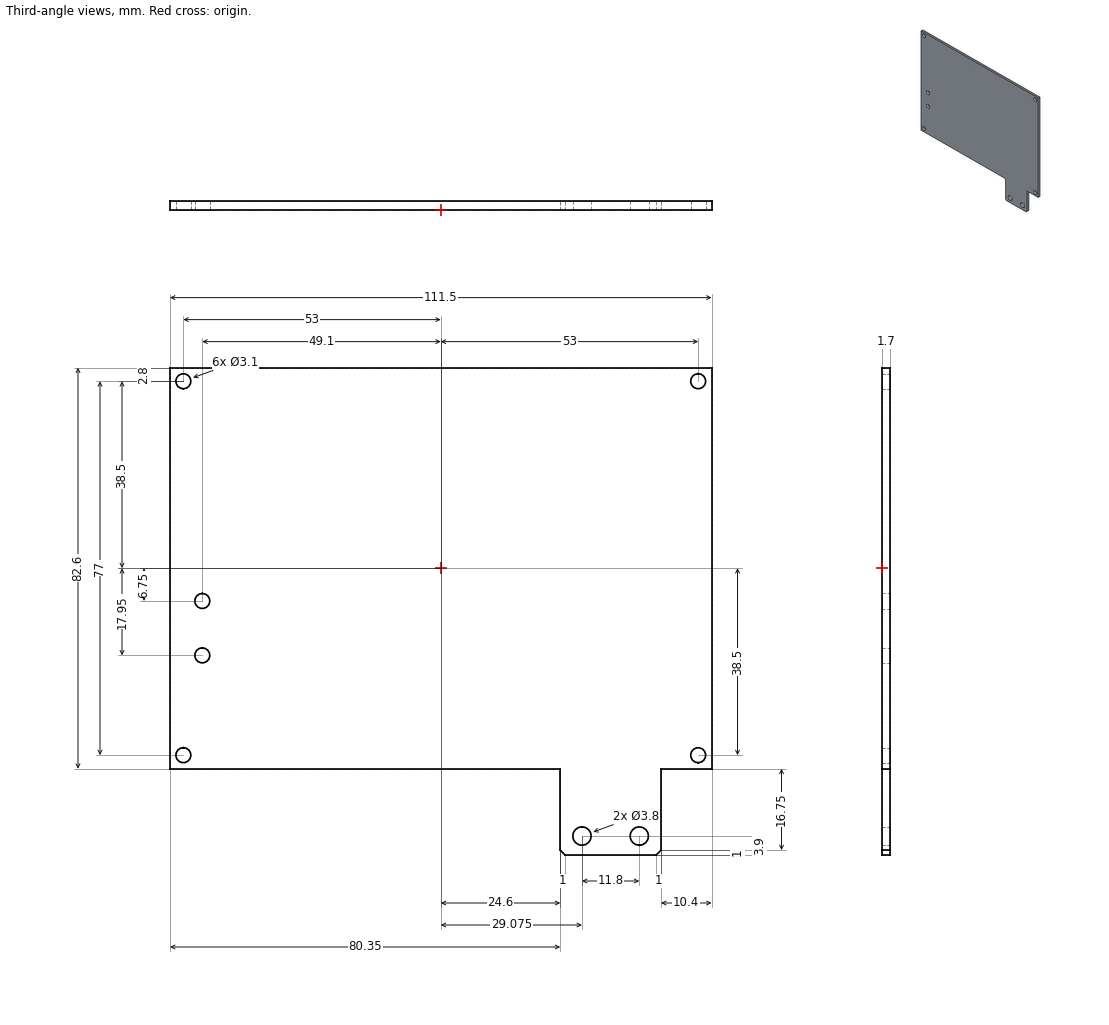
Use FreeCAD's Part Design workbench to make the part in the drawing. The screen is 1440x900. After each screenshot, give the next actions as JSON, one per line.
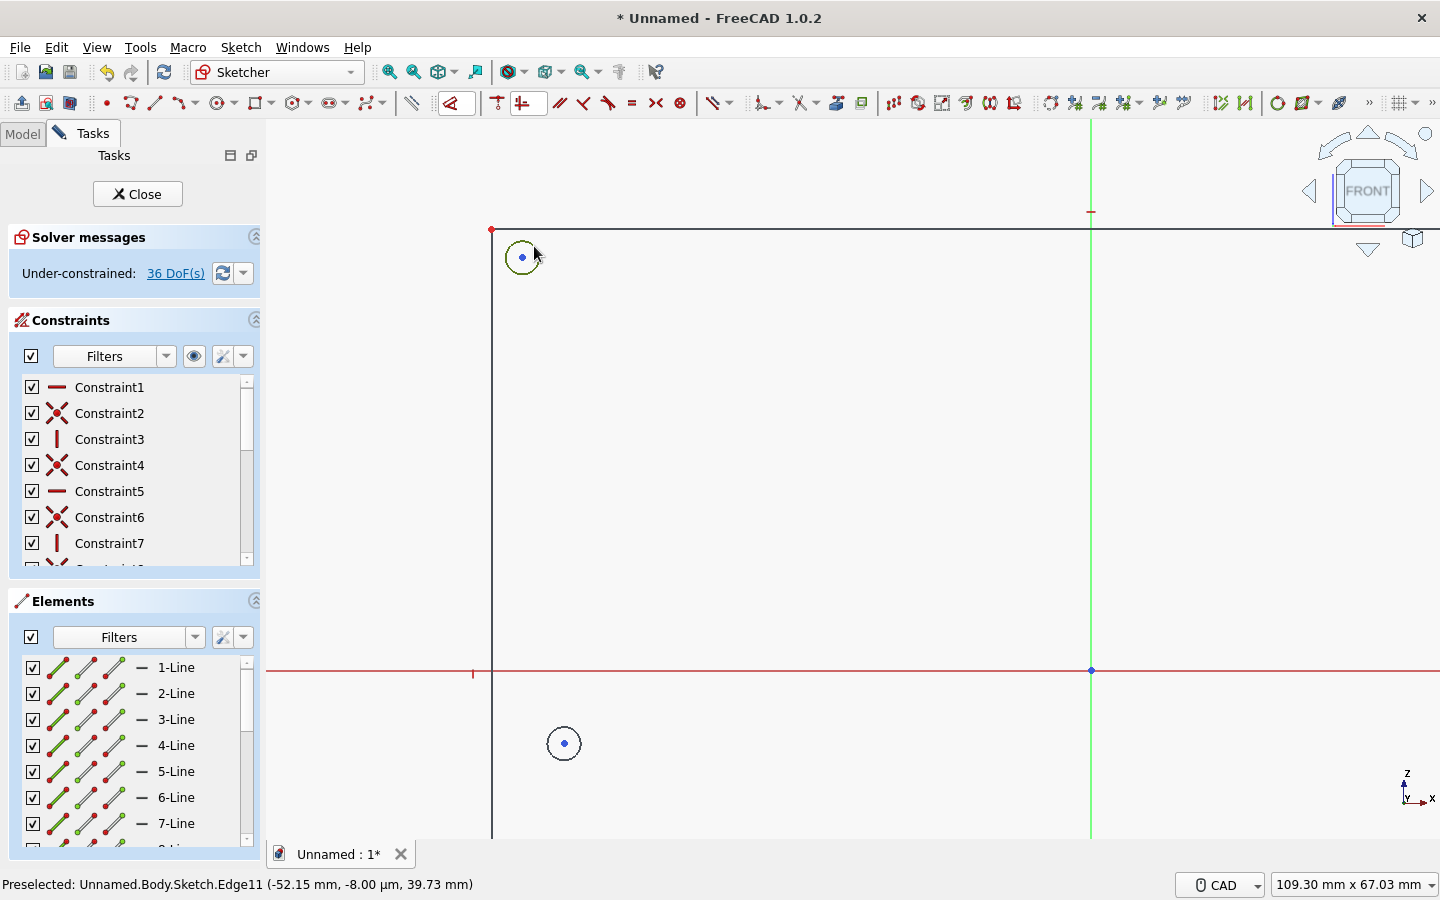
{"action": "left_click", "coordinate": [576, 732]}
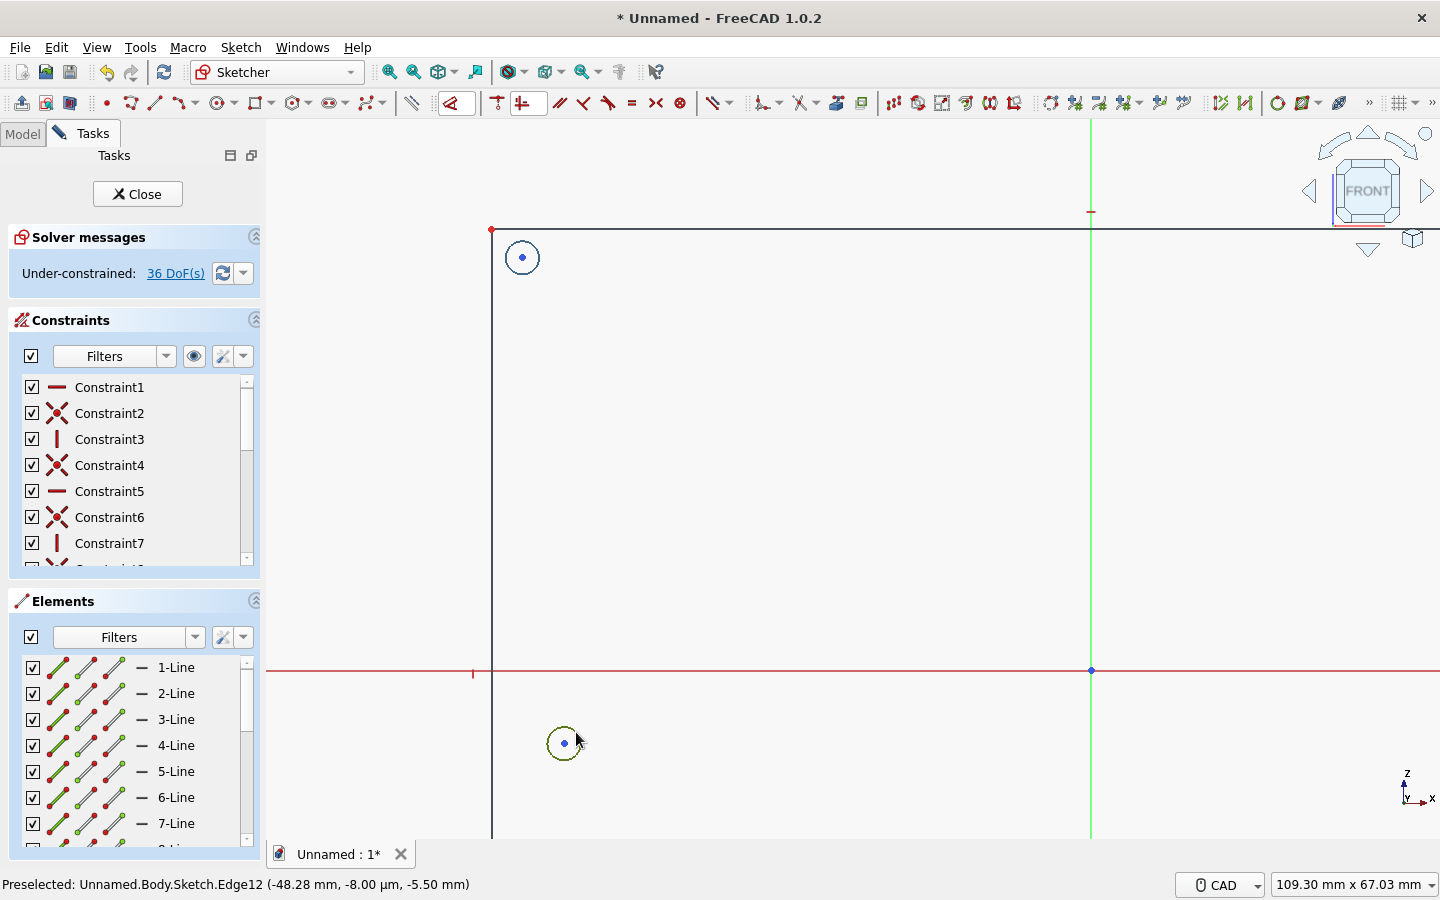
{"action": "scroll", "coordinate": [534, 245], "scroll_direction": "down", "scroll_amount": 4}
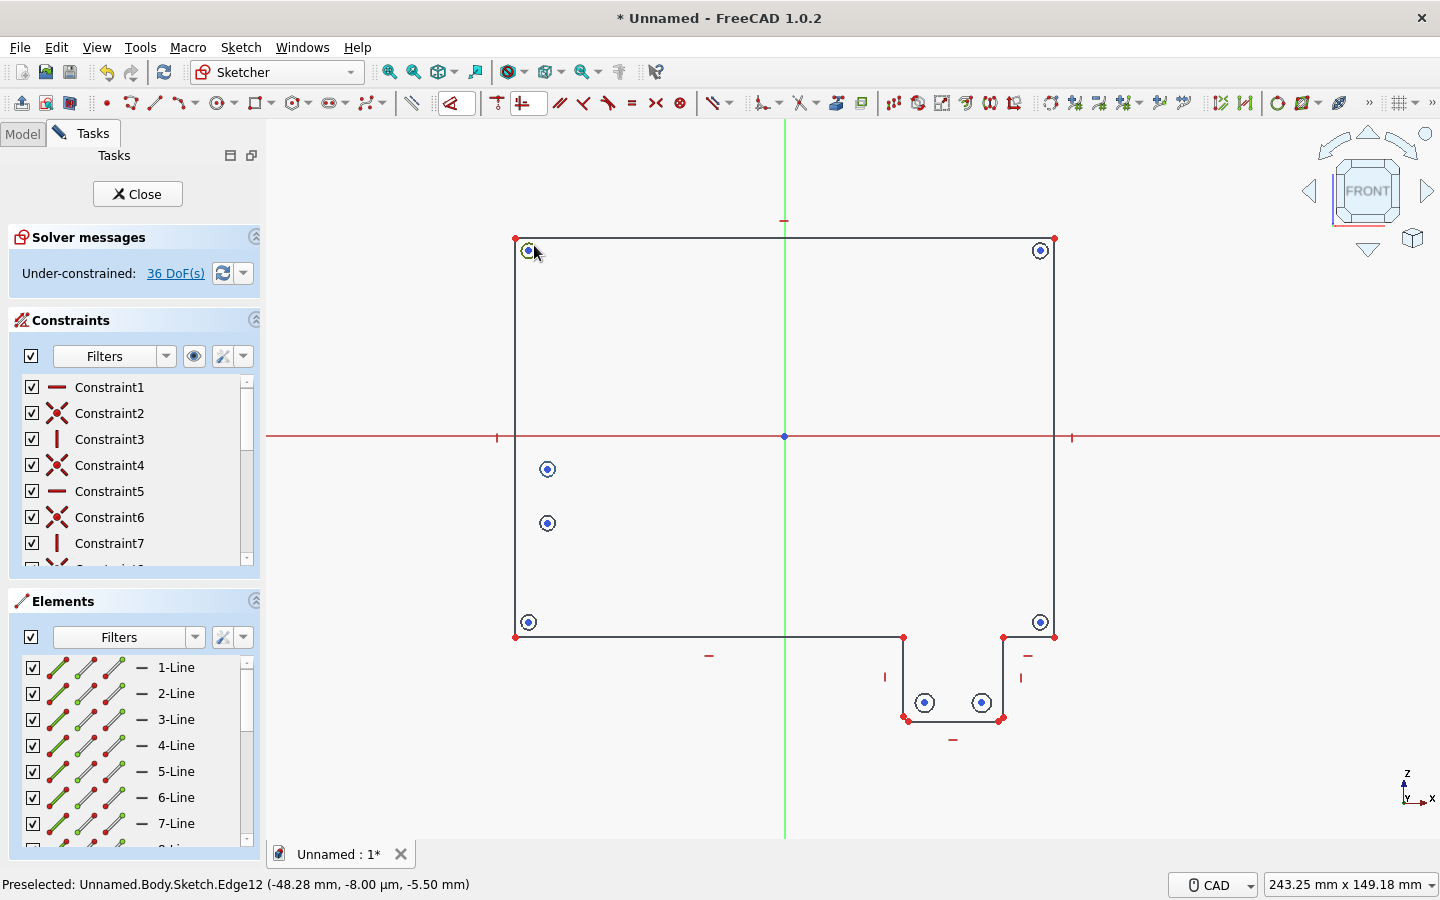
{"action": "scroll", "coordinate": [1046, 245], "scroll_direction": "up", "scroll_amount": 4}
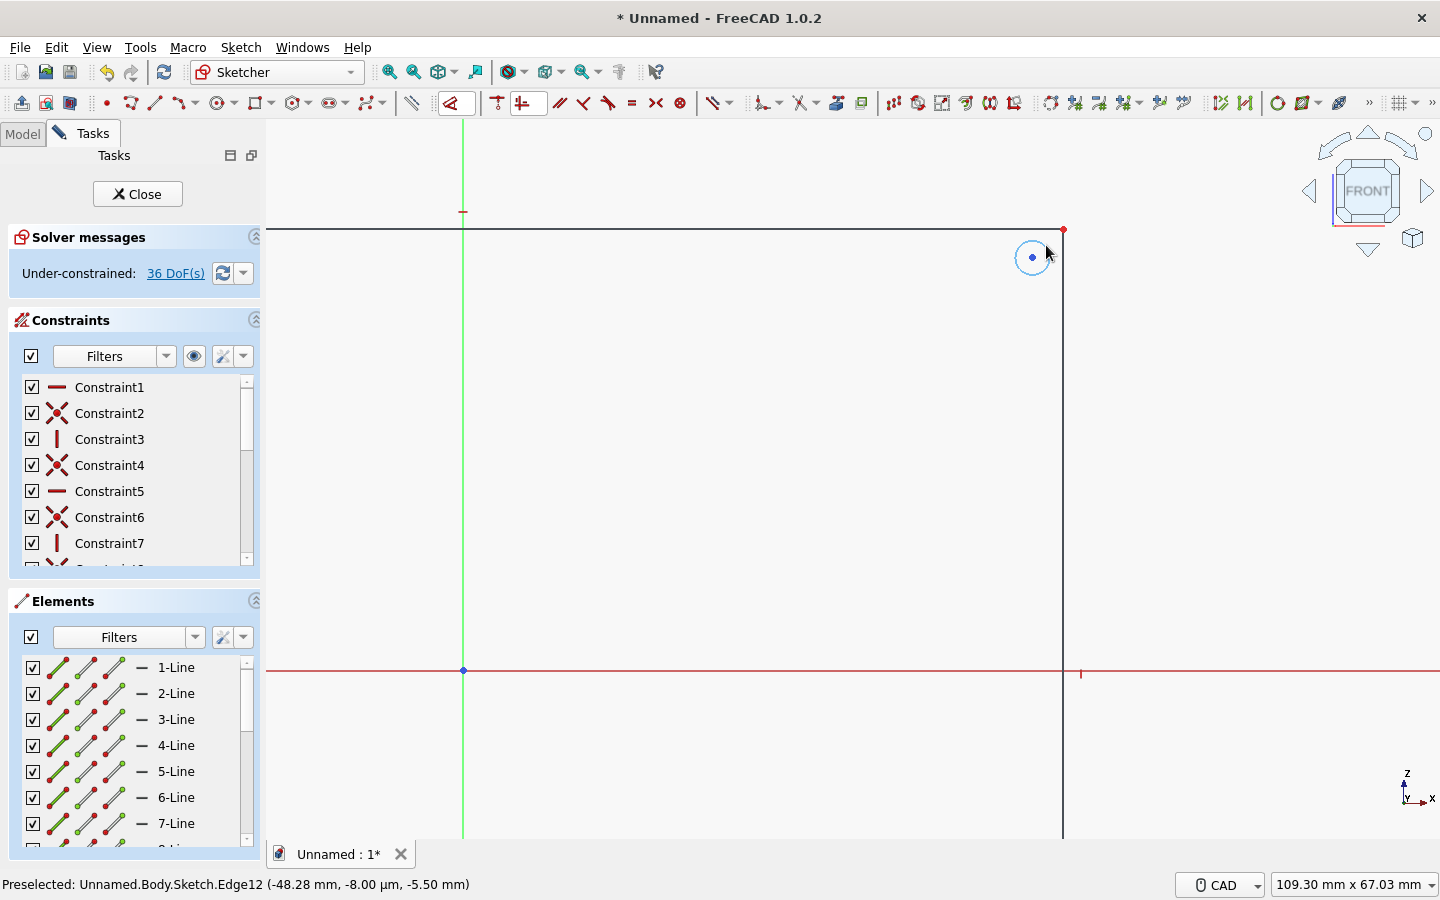
{"action": "left_click", "coordinate": [1045, 246]}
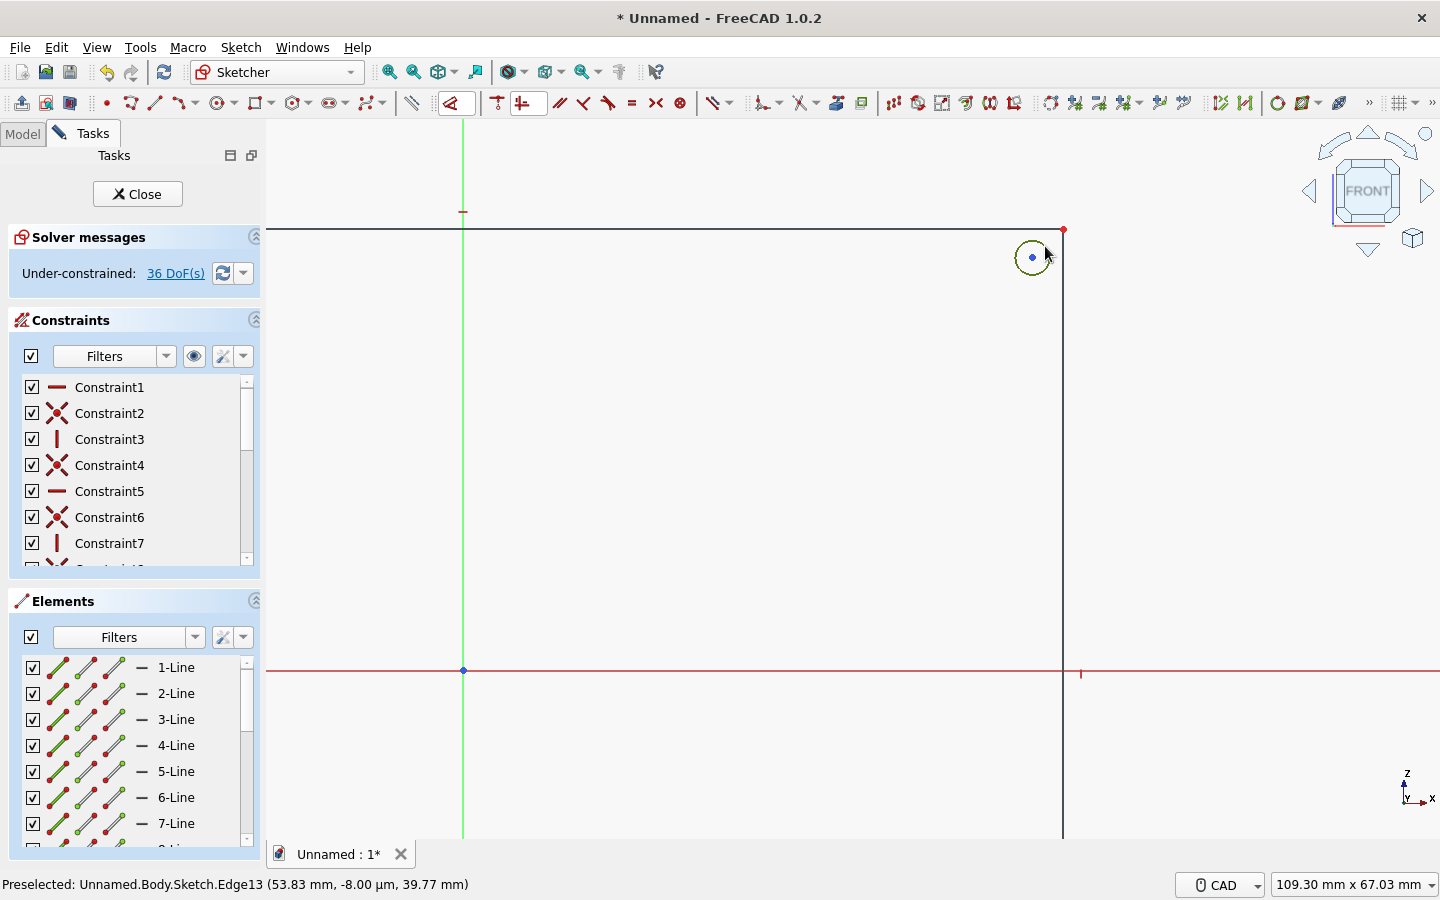
{"action": "scroll", "coordinate": [1046, 245], "scroll_direction": "down", "scroll_amount": 4}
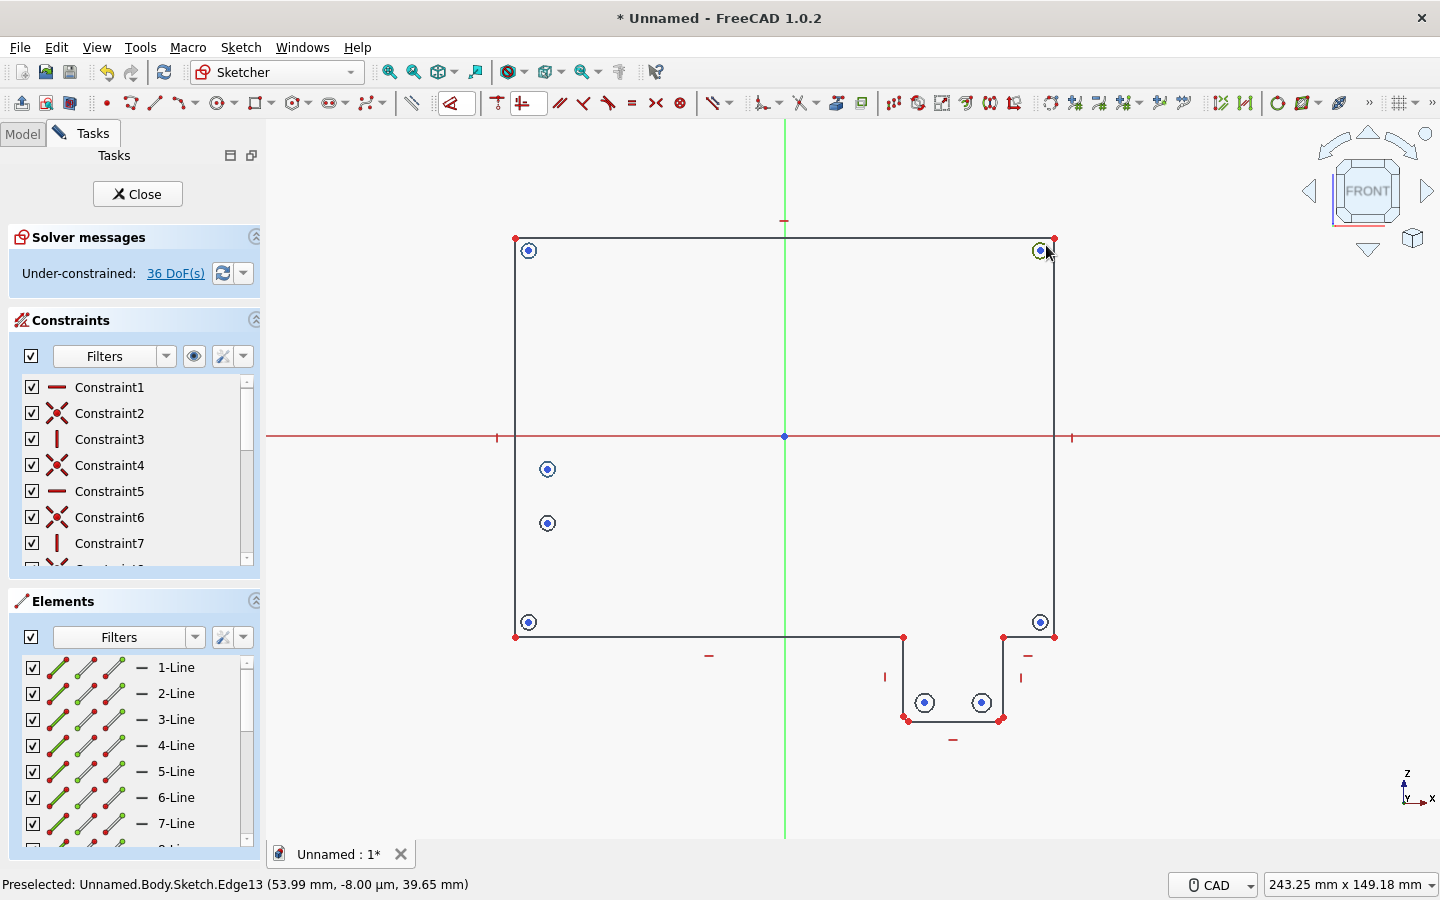
{"action": "scroll", "coordinate": [553, 518], "scroll_direction": "up", "scroll_amount": 4}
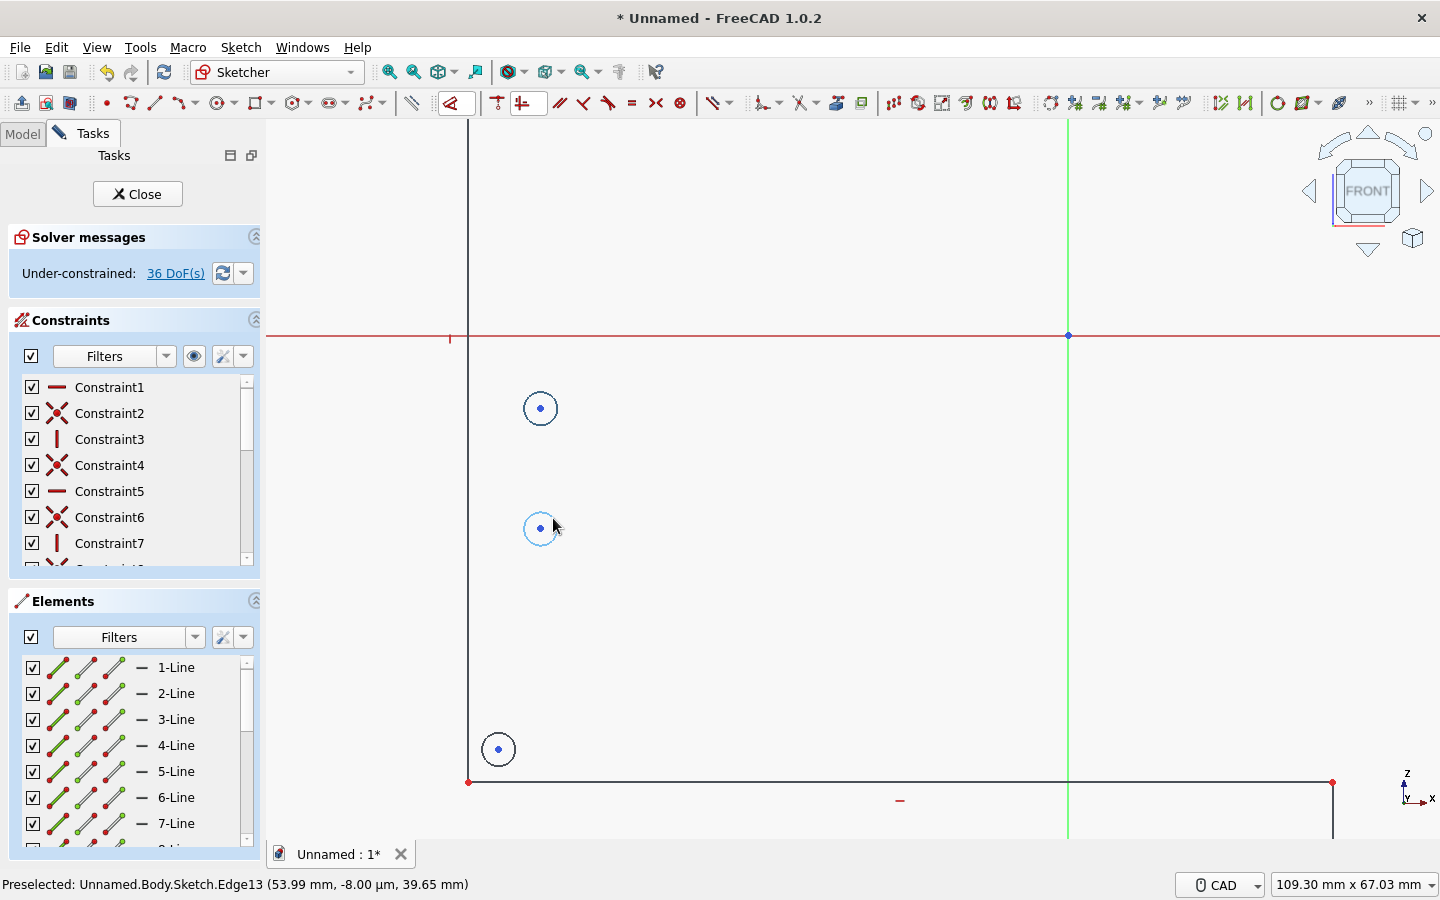
{"action": "left_click", "coordinate": [552, 517]}